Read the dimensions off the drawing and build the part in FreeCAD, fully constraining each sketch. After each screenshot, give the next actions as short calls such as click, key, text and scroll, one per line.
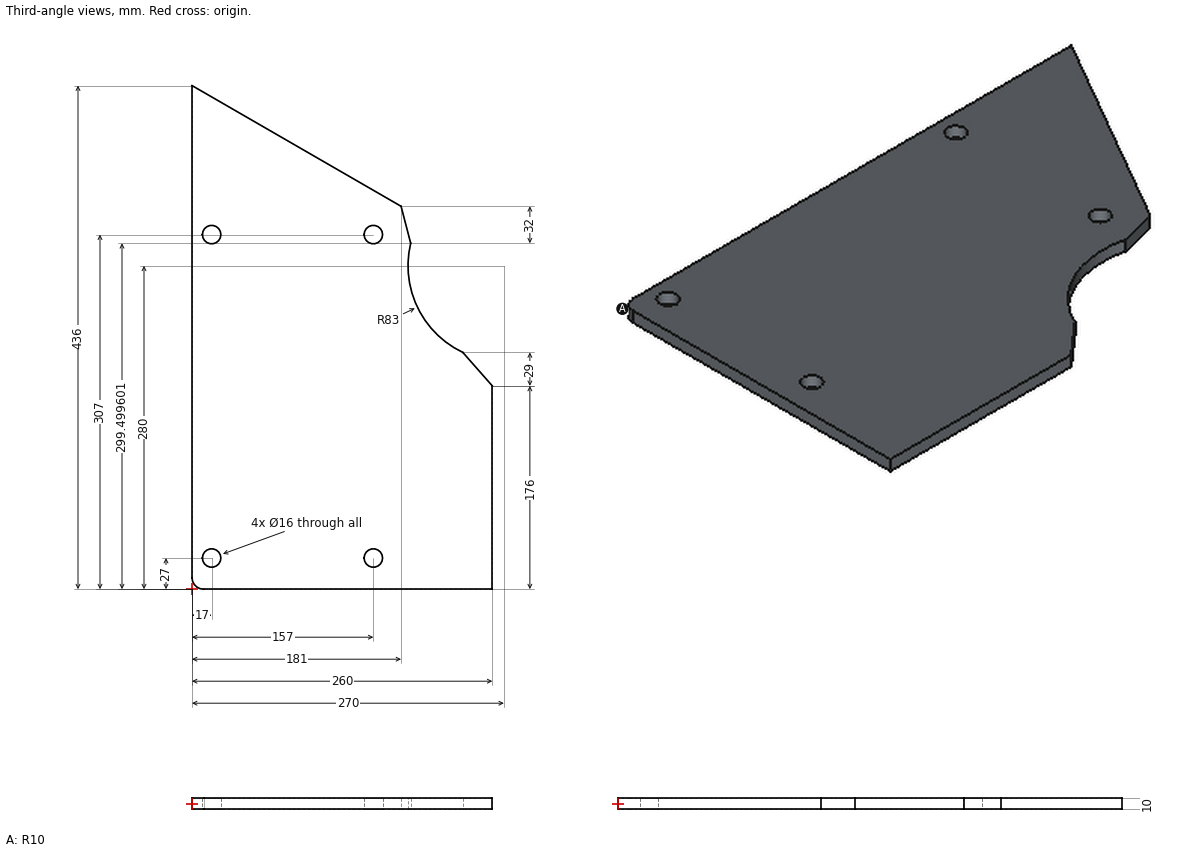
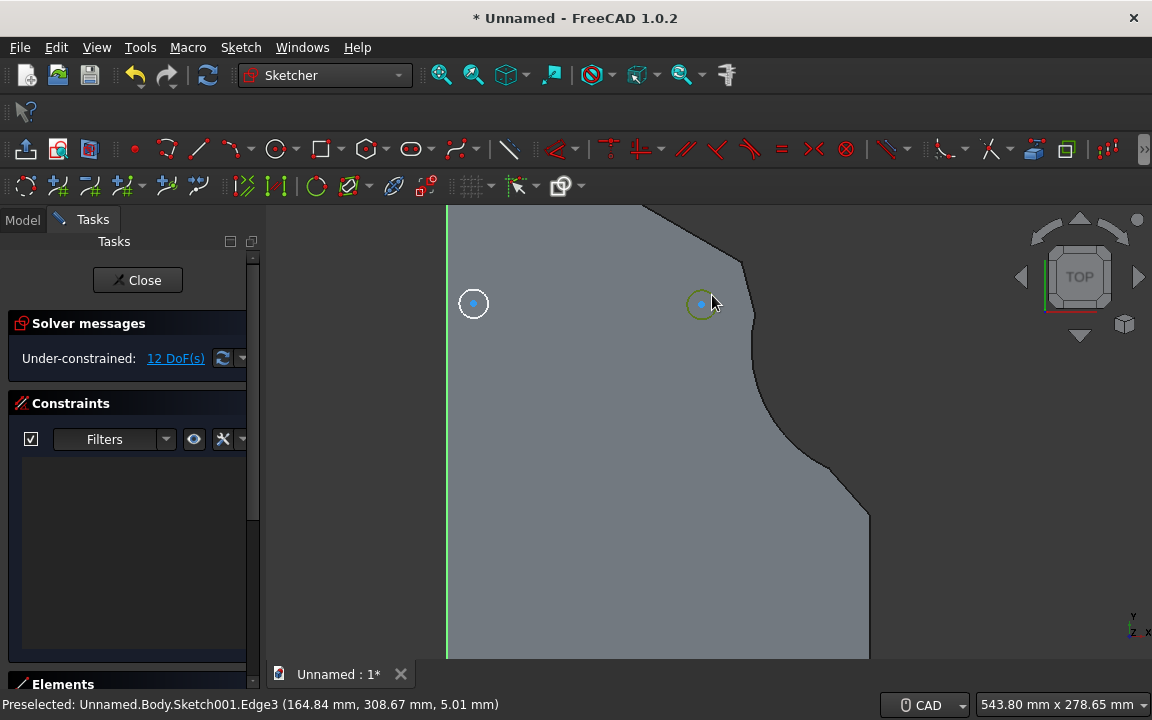
click(484, 294)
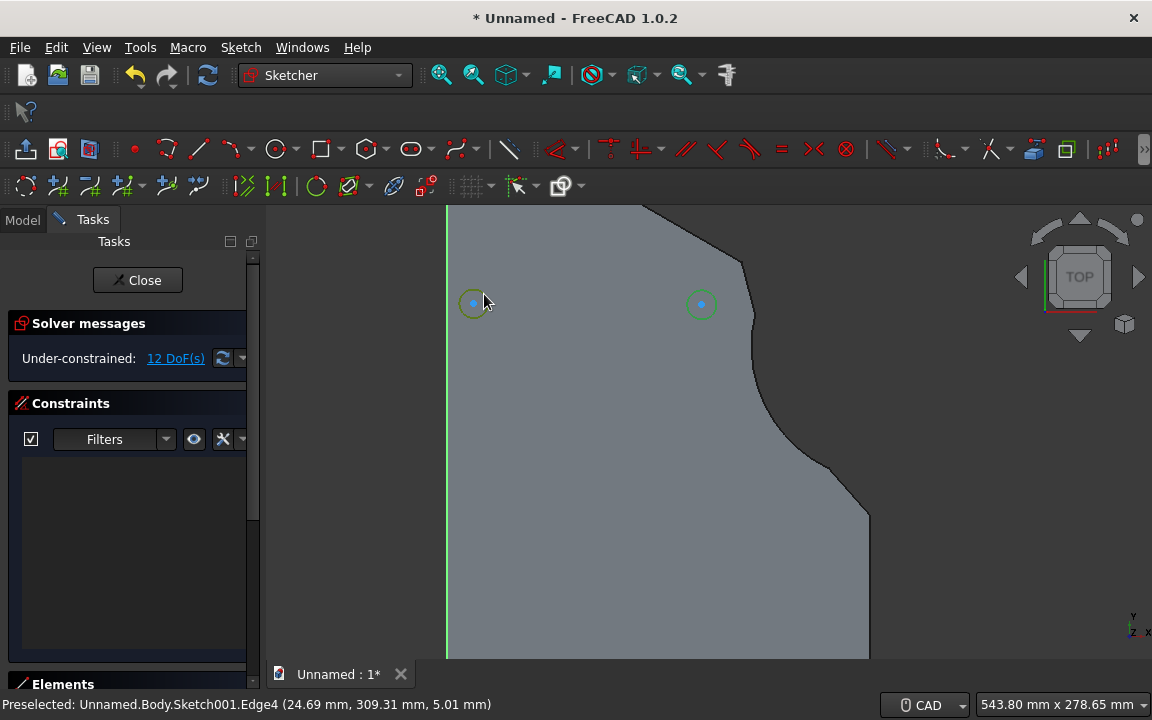
key(e)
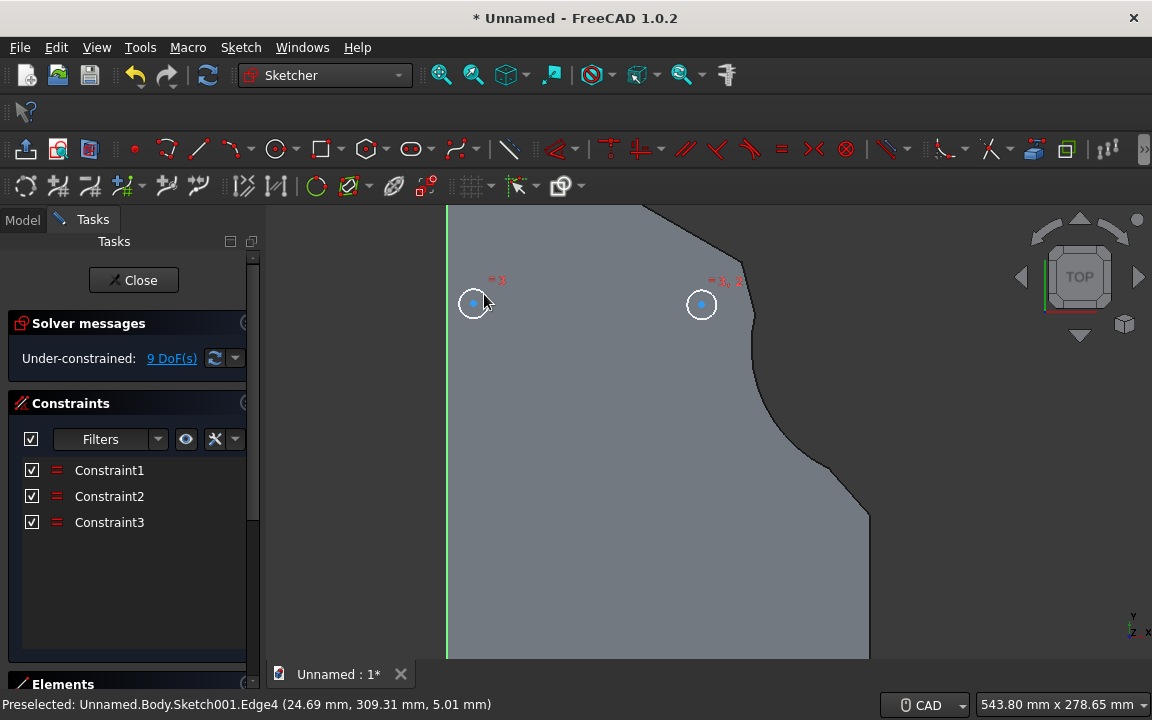
key(d)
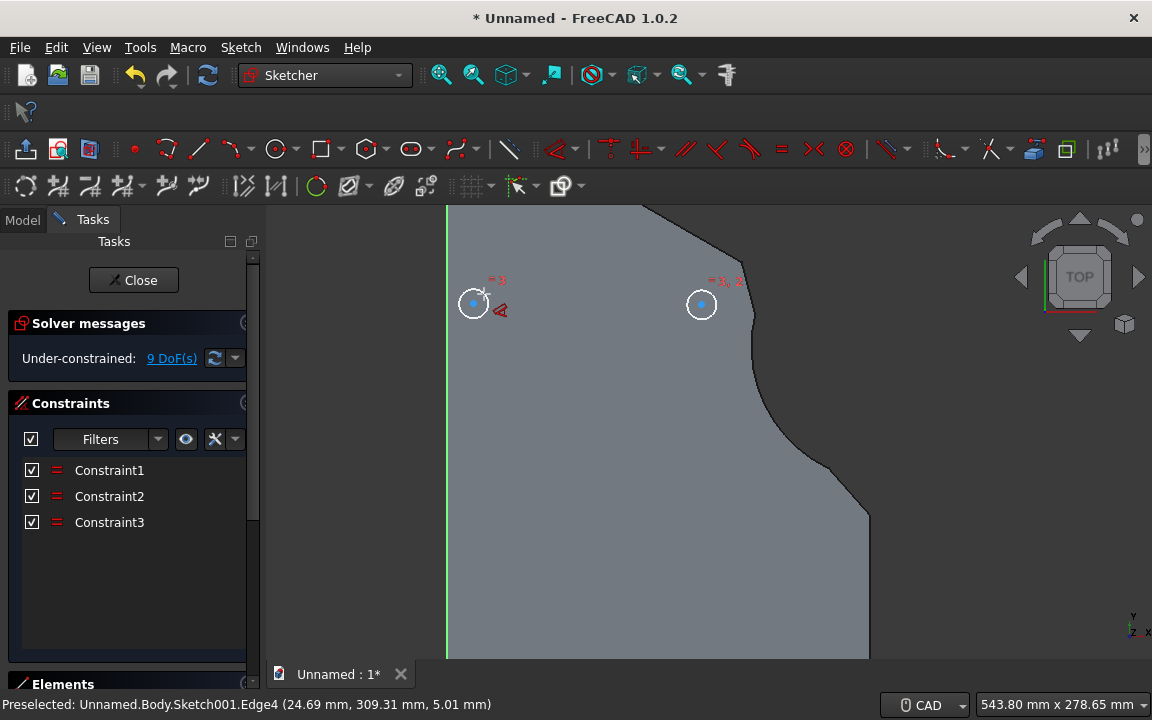
scroll(713, 294, down, 3)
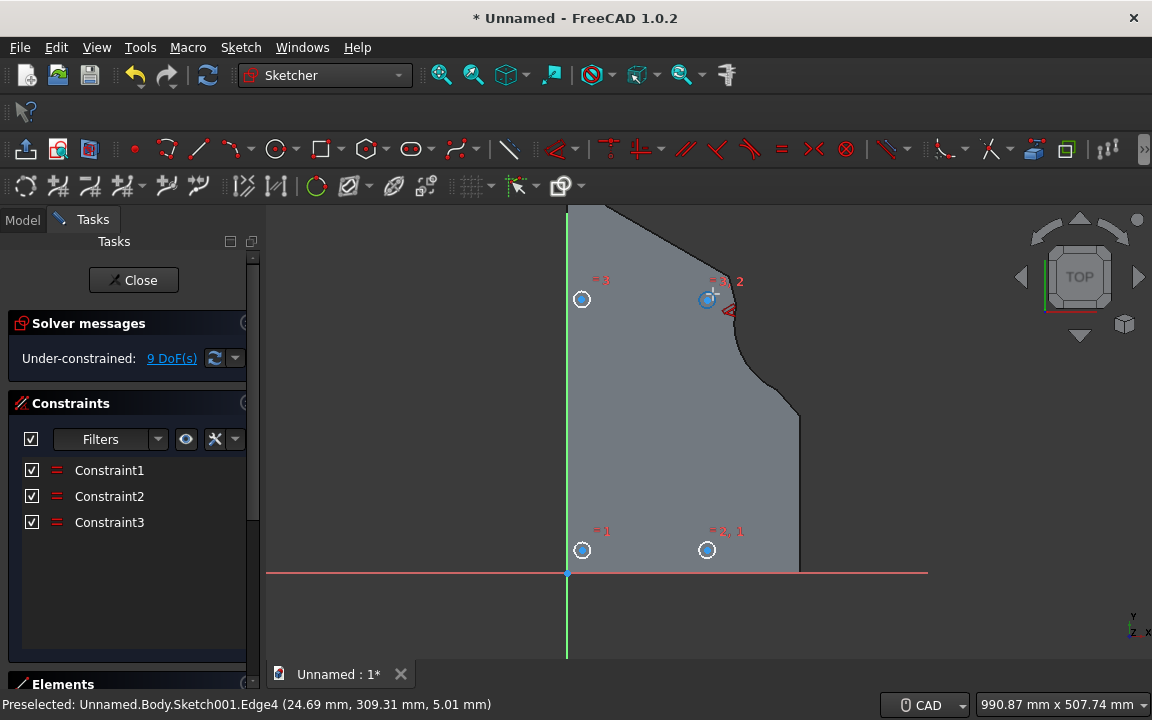
scroll(588, 545, up, 6)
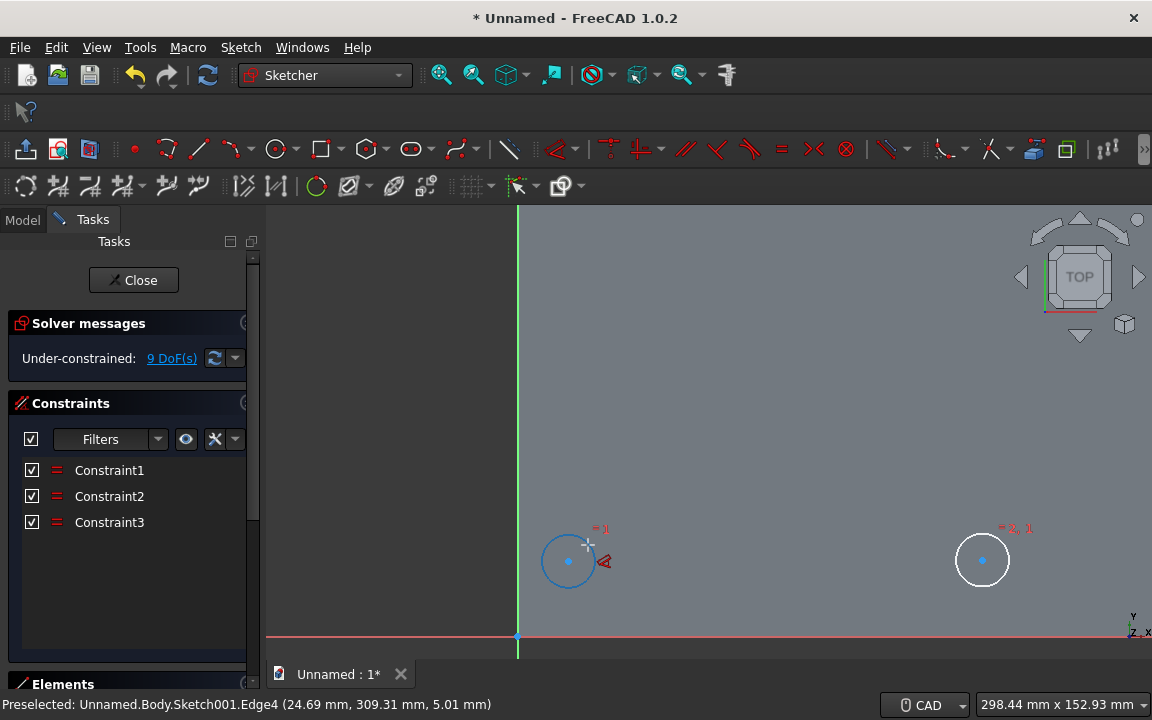
click(587, 543)
click(610, 521)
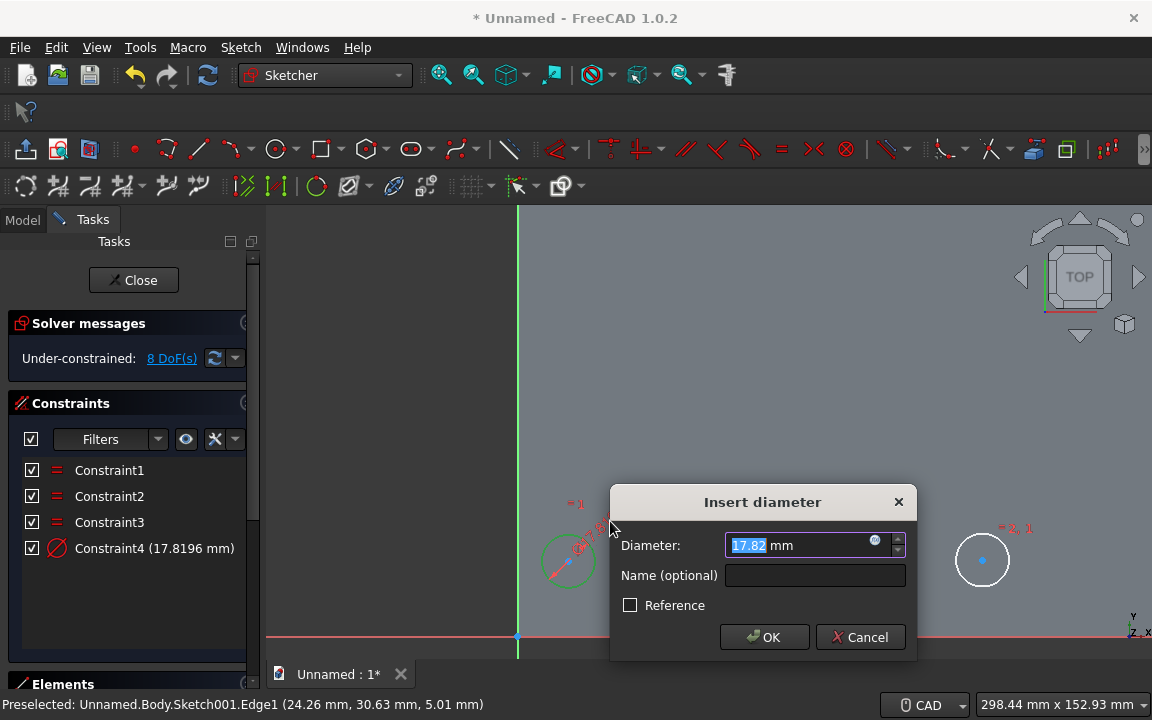
text(16)
key(Return)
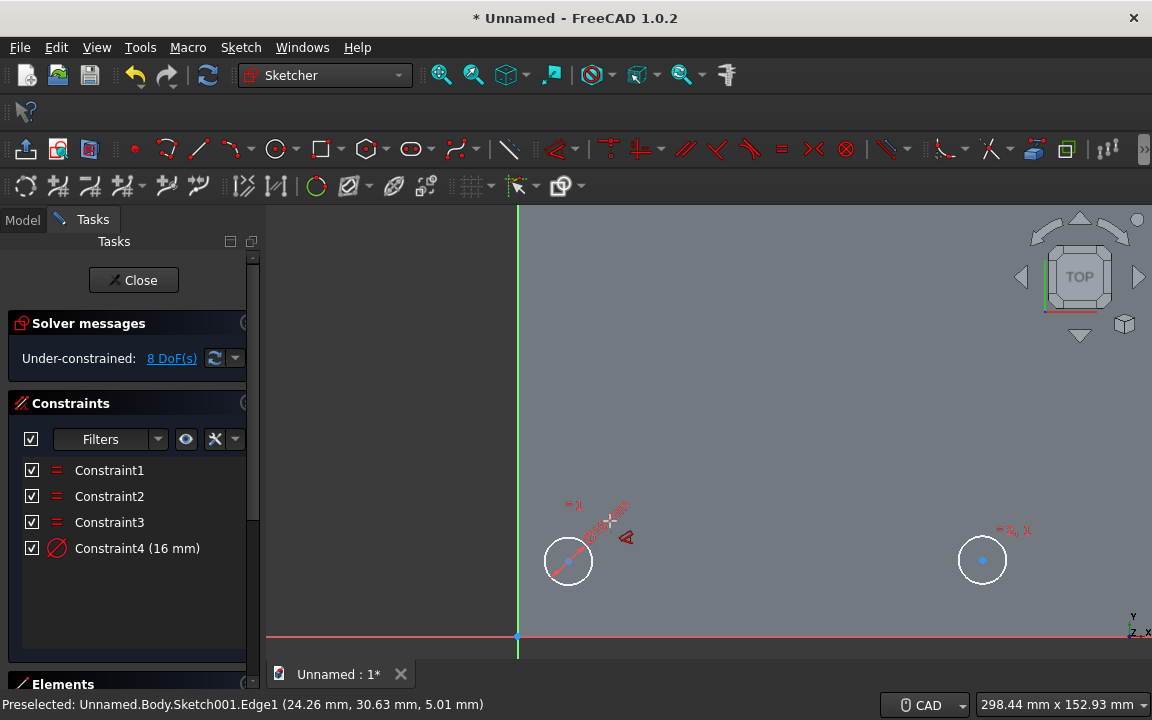
click(568, 561)
click(531, 527)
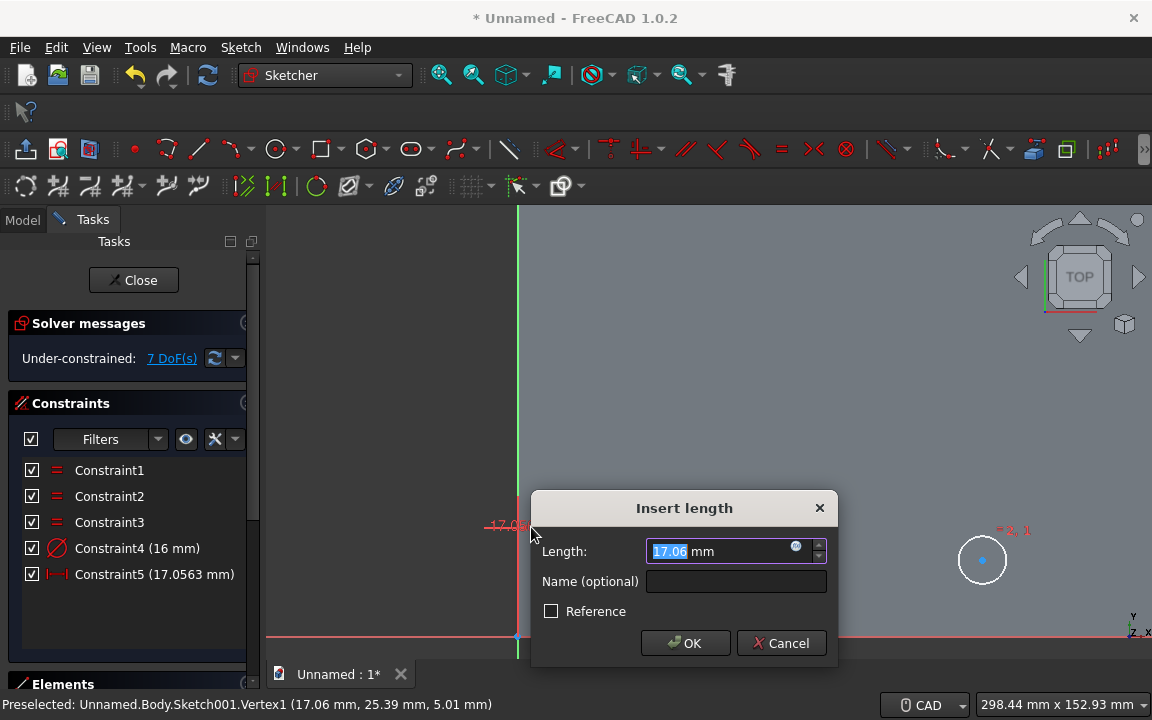
text(17)
key(Return)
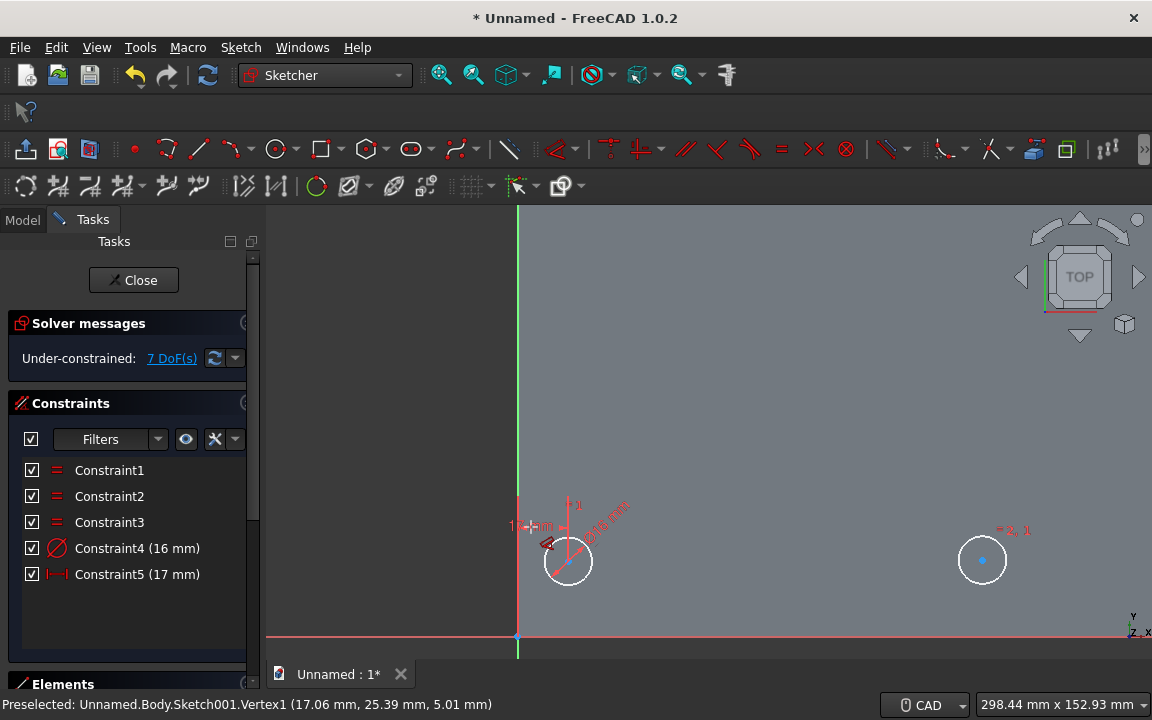
click(568, 561)
click(484, 596)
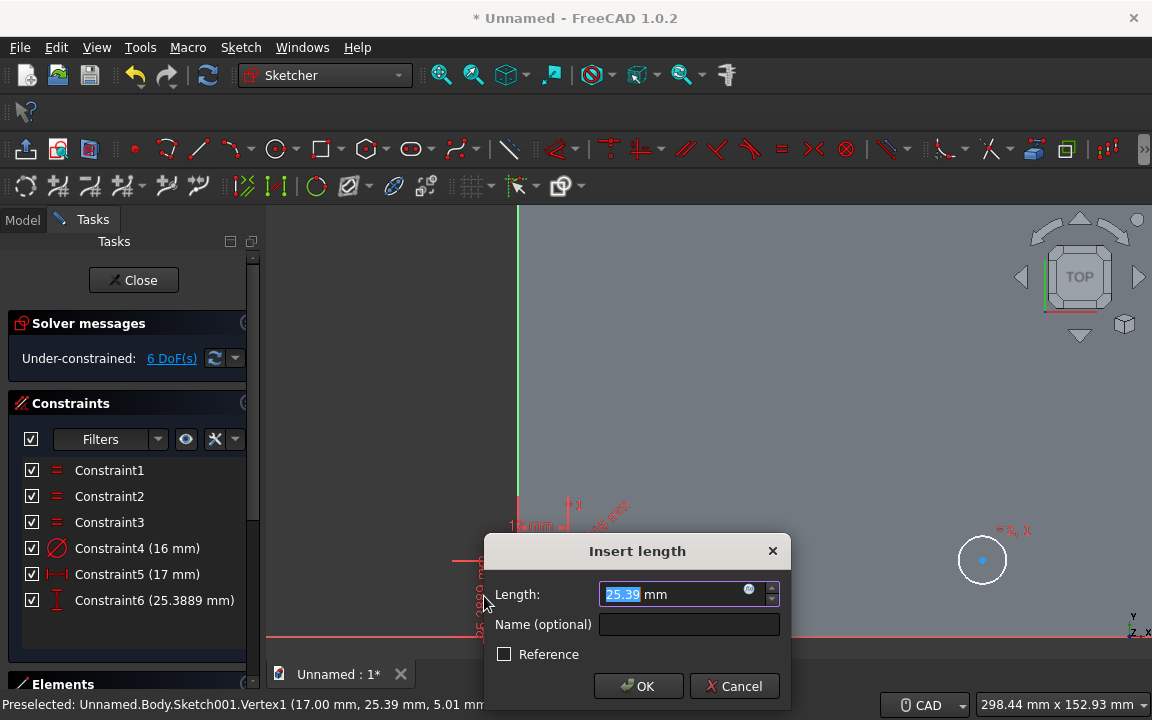
text(27)
key(Return)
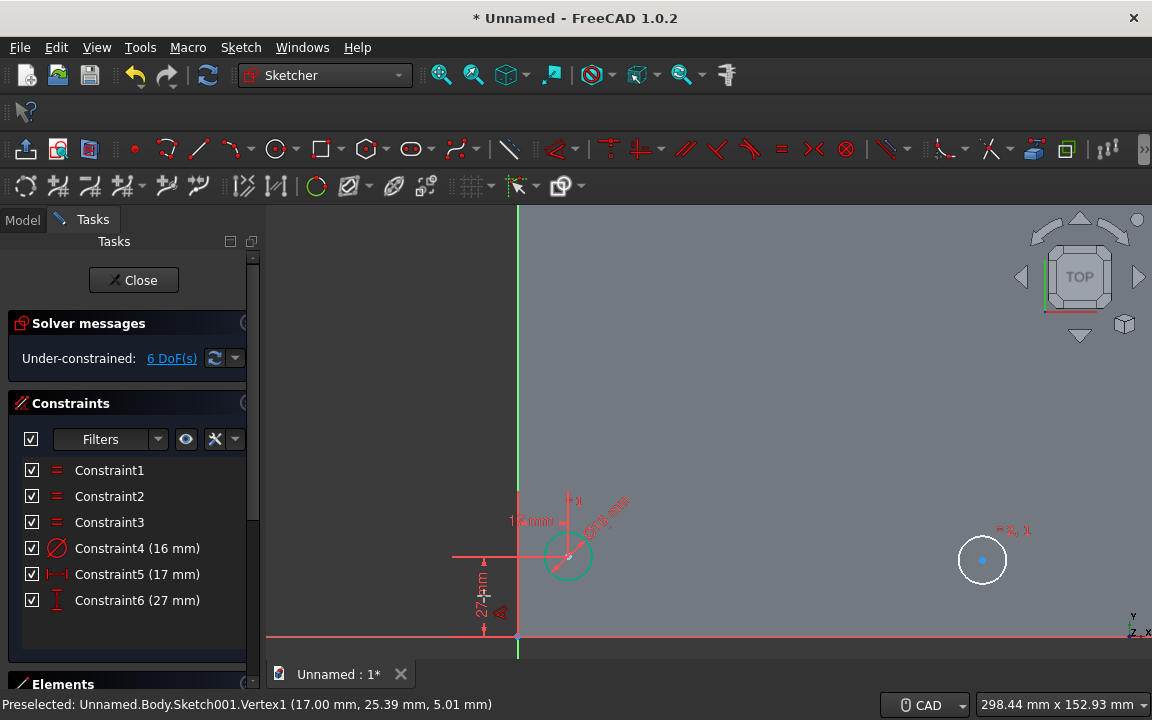
click(983, 560)
click(484, 571)